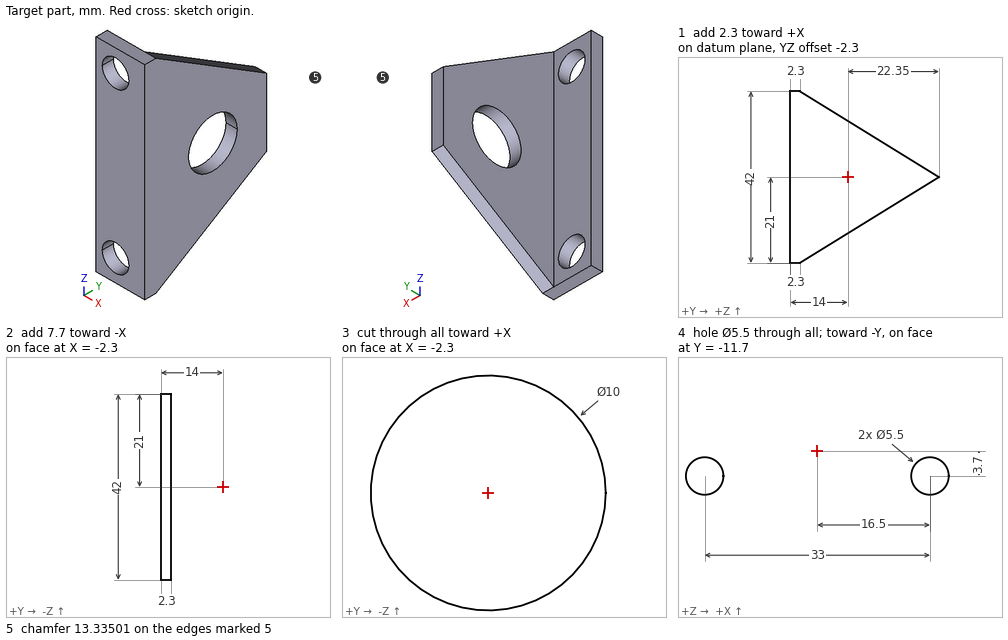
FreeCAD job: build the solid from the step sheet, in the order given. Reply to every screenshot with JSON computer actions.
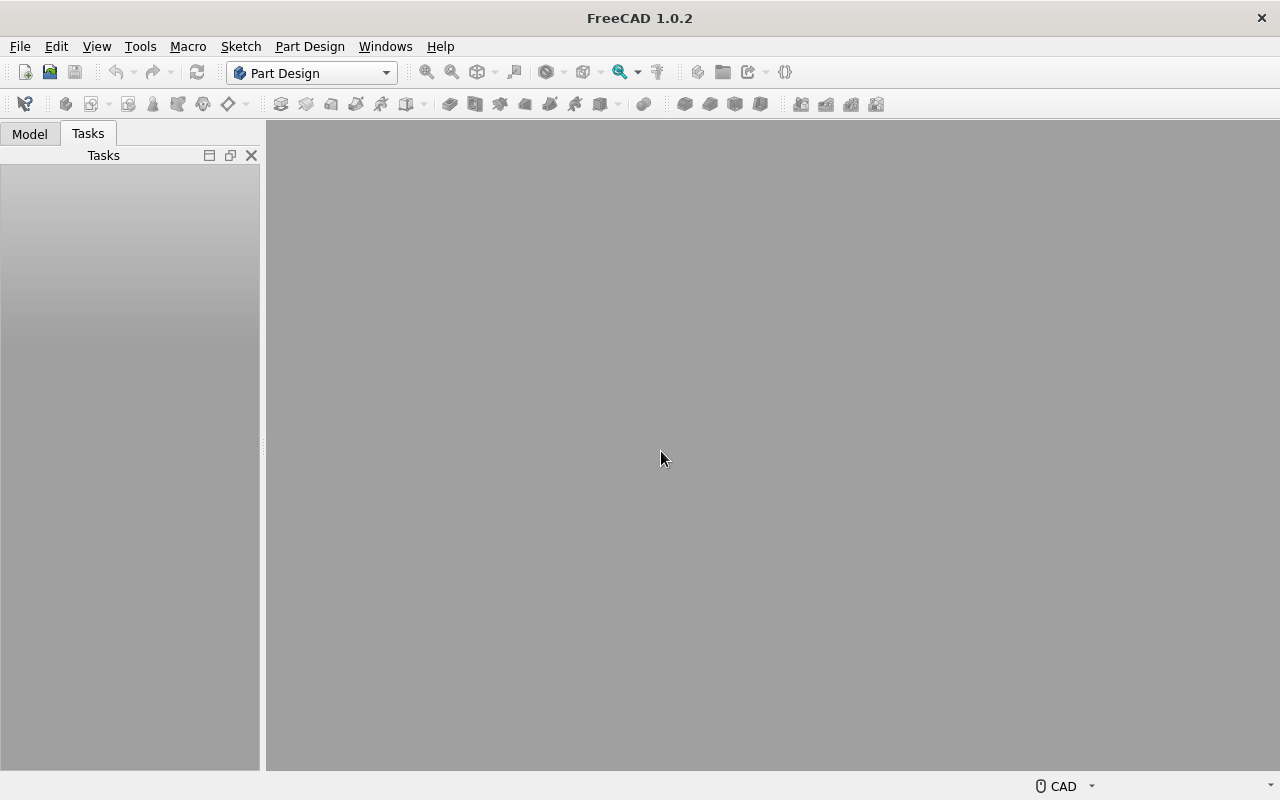
{"action": "key", "text": "ctrl+n"}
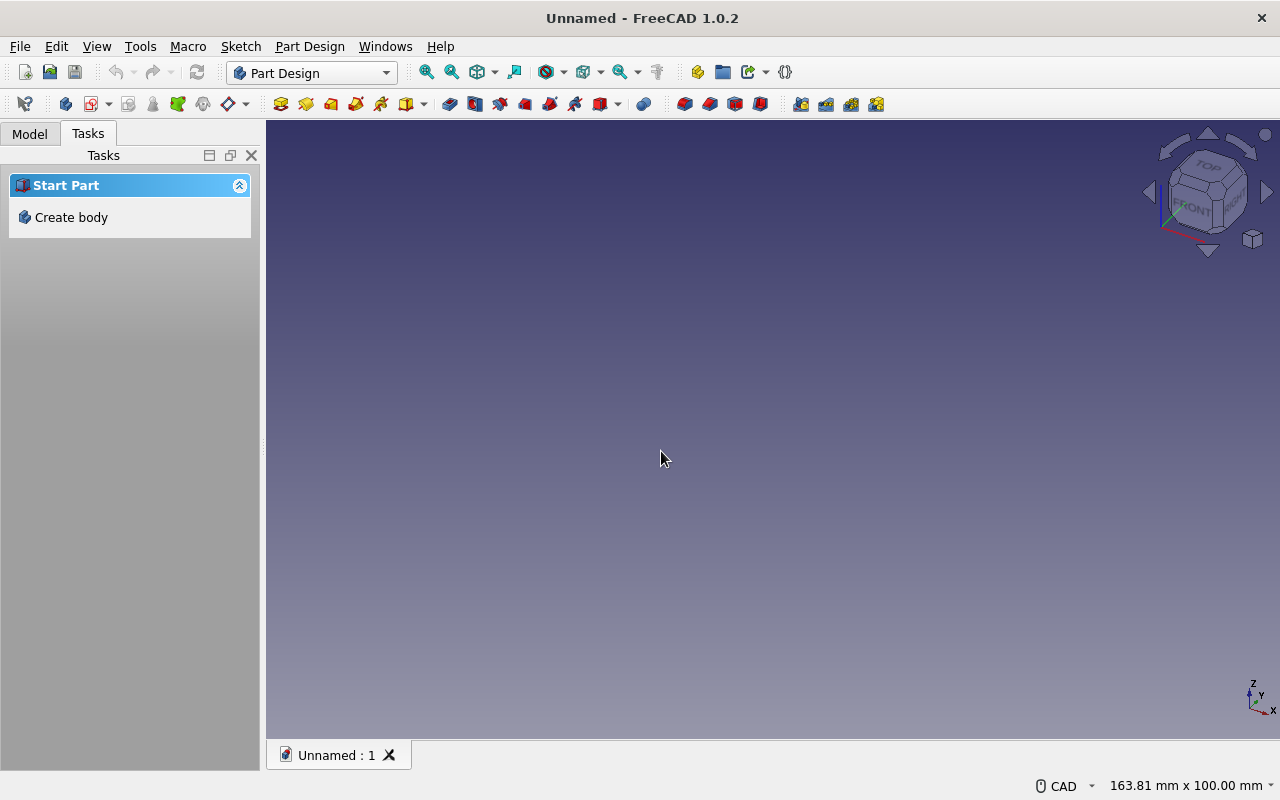
{"action": "left_click", "coordinate": [66, 104]}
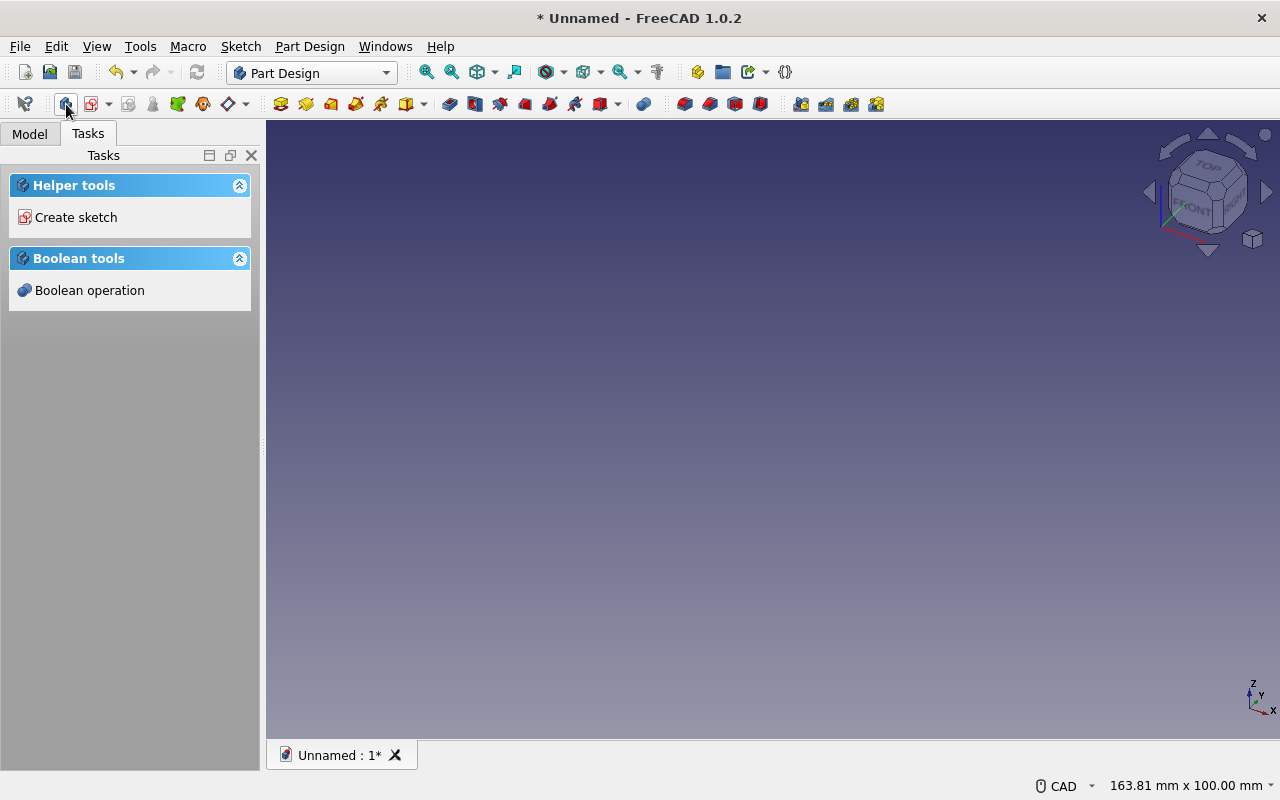
{"action": "left_click", "coordinate": [30, 134]}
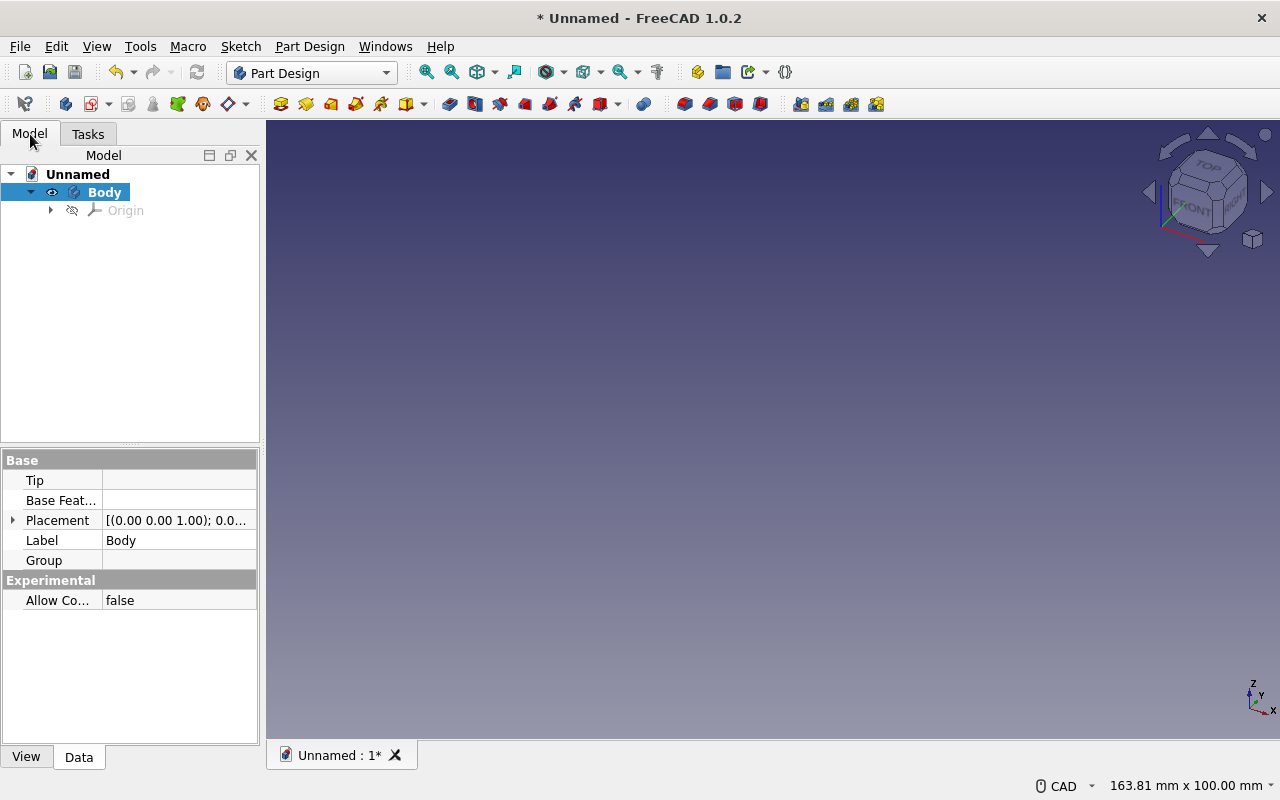
{"action": "left_click", "coordinate": [51, 210]}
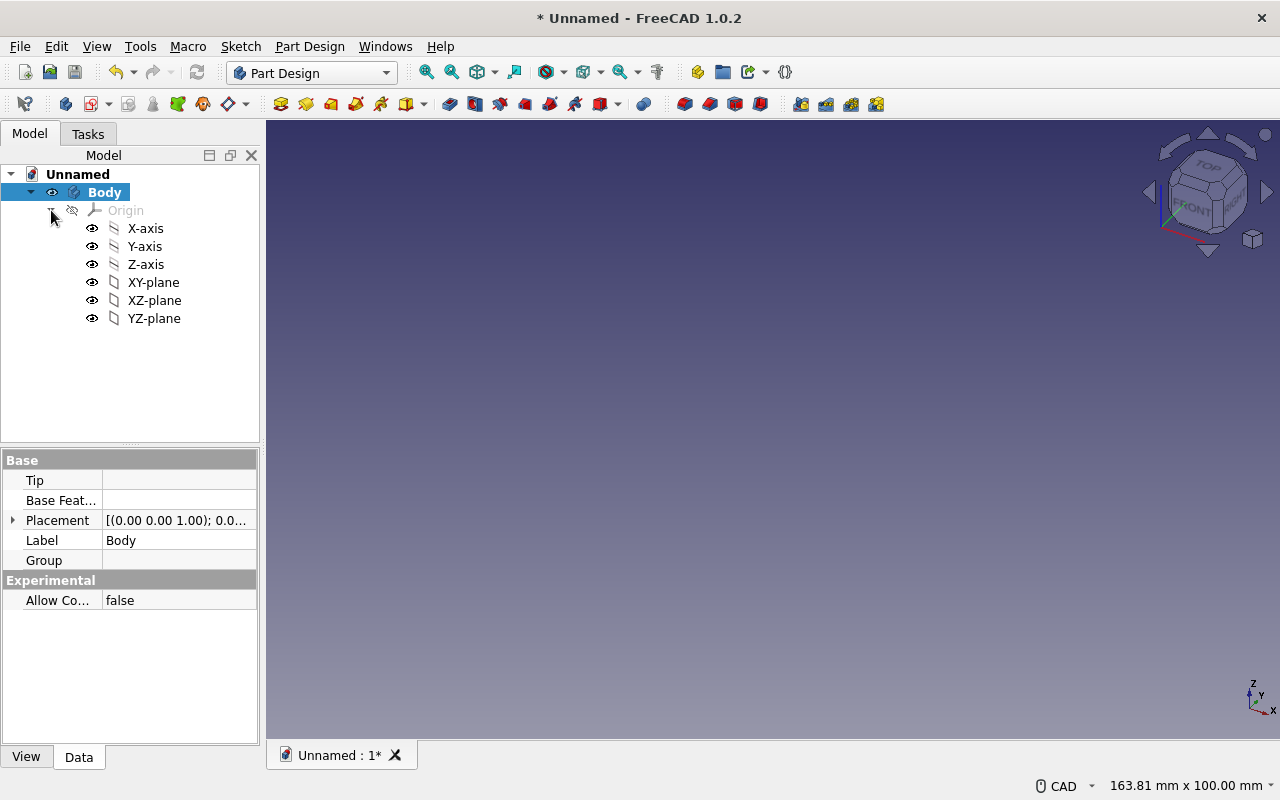
{"action": "left_click", "coordinate": [137, 318]}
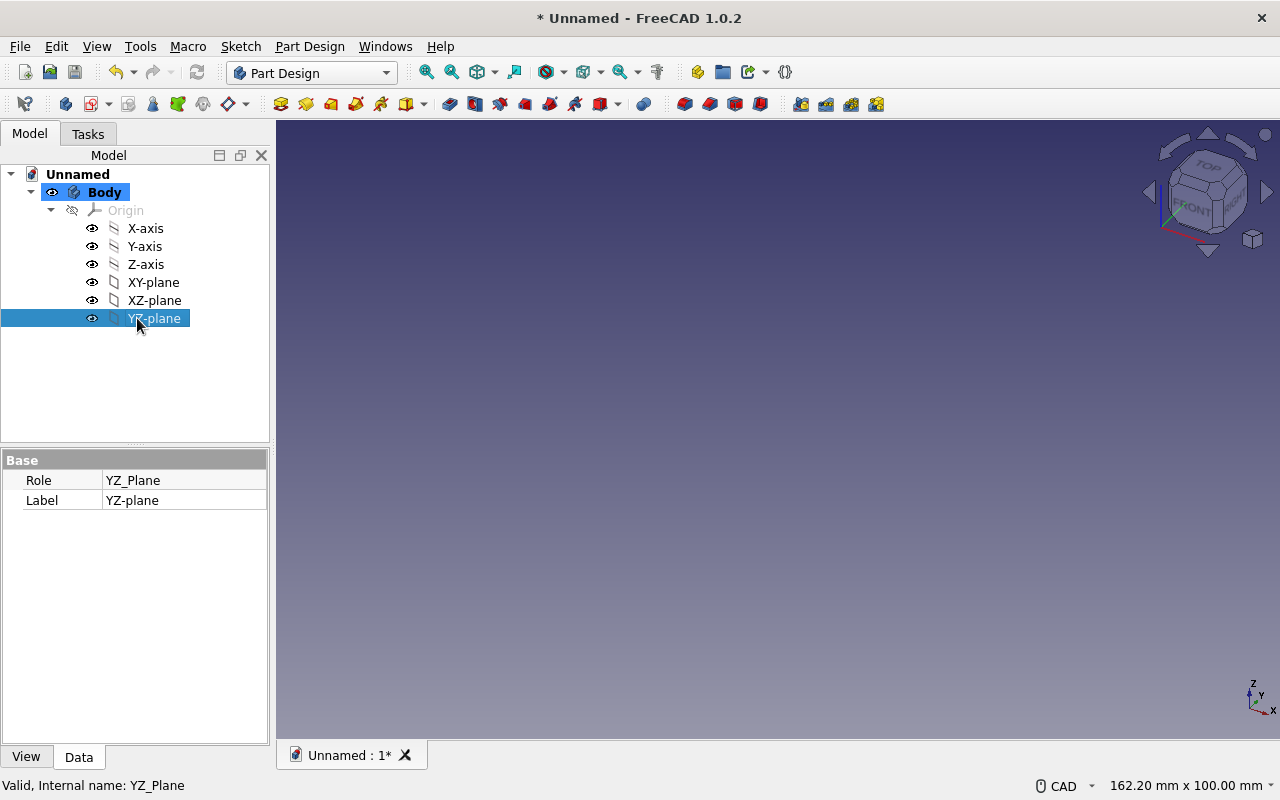
{"action": "left_click", "coordinate": [228, 104]}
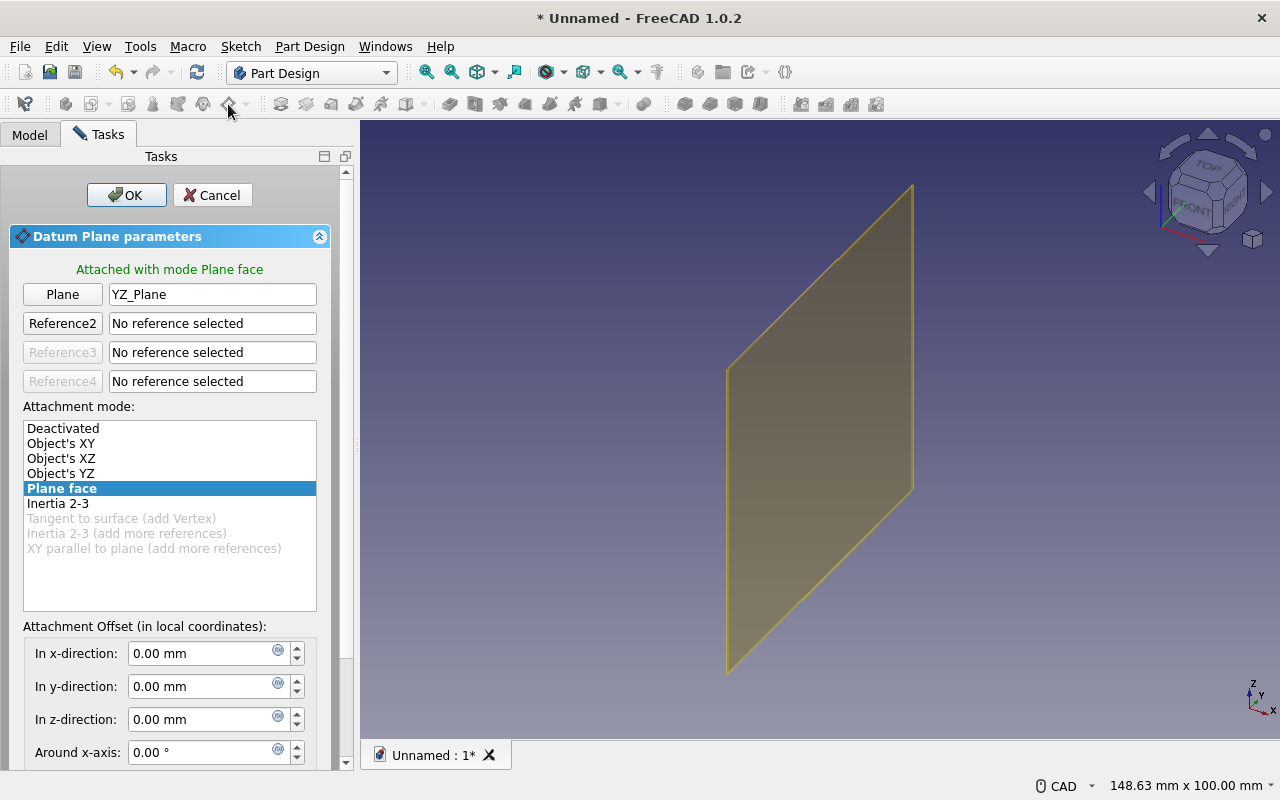
{"action": "triple_click", "coordinate": [210, 720]}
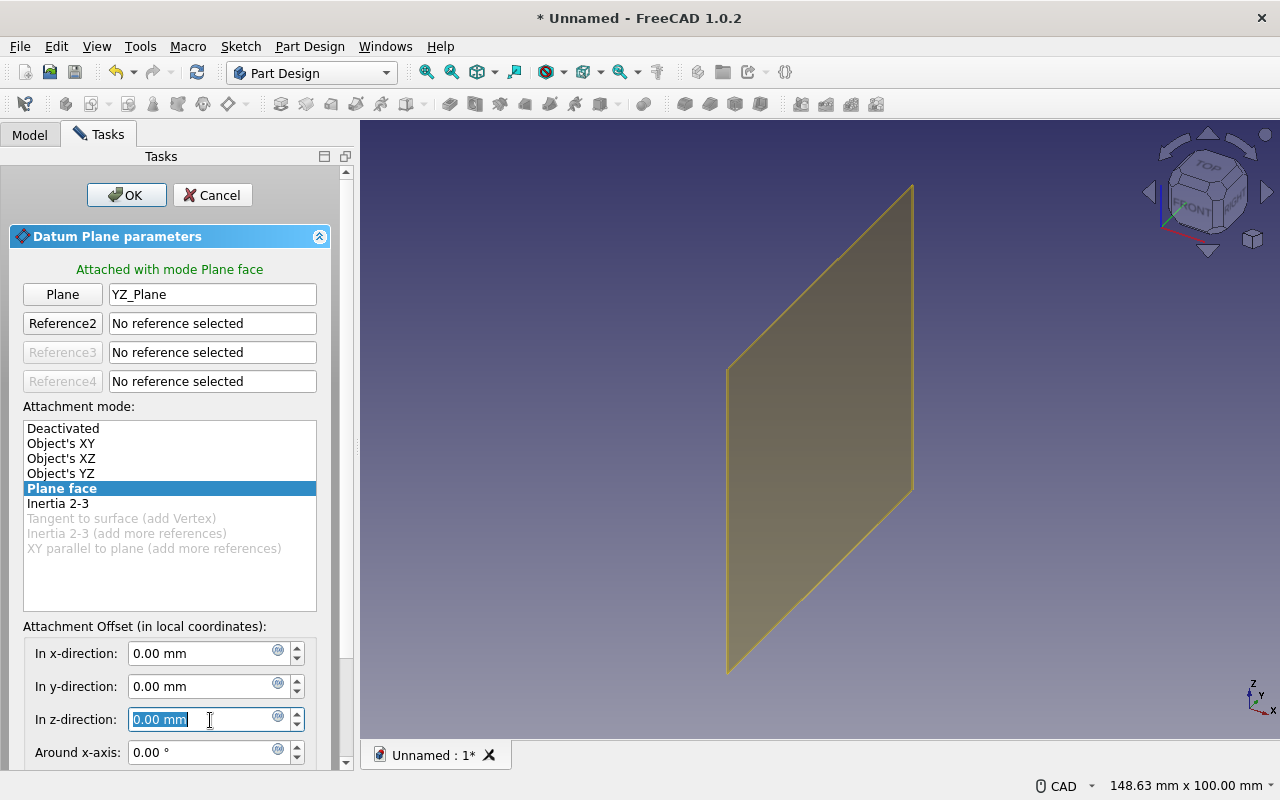
{"action": "type", "text": "-2.3"}
{"action": "key", "text": "Tab"}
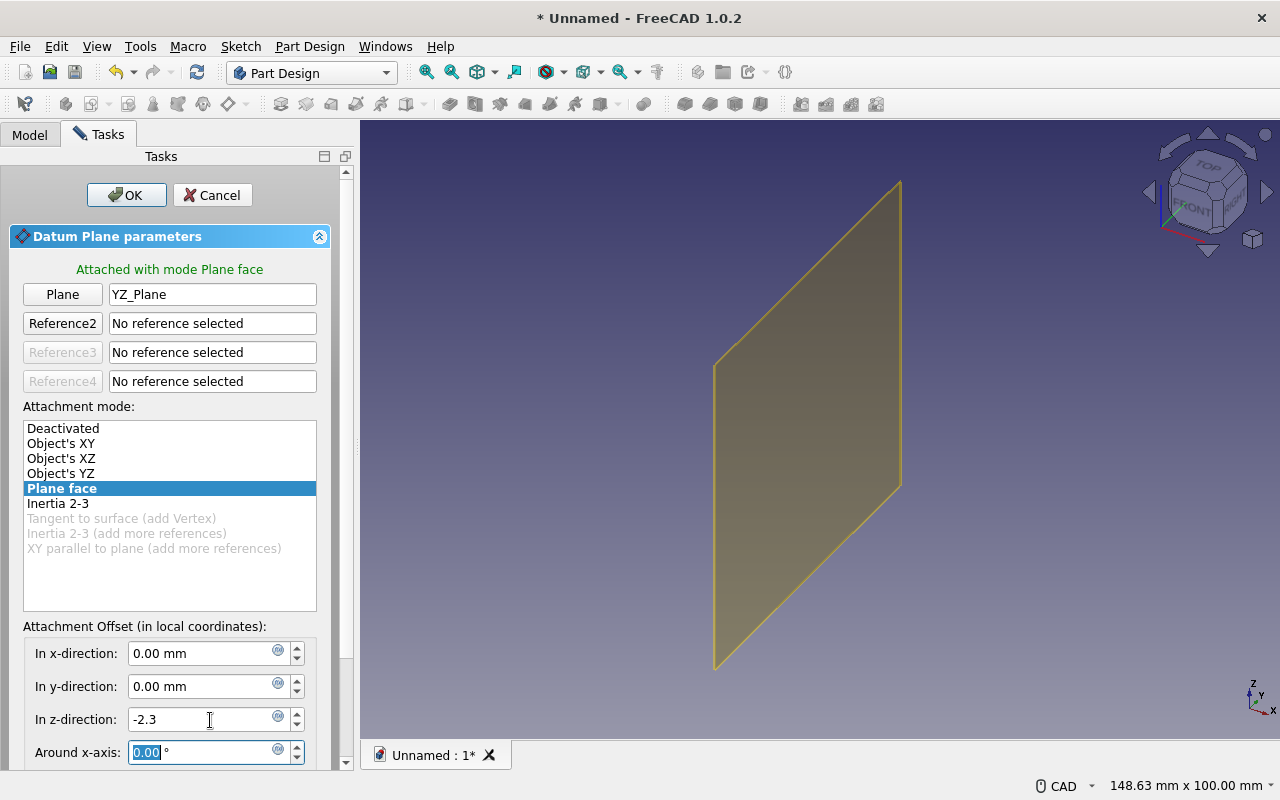
{"action": "left_click", "coordinate": [127, 195]}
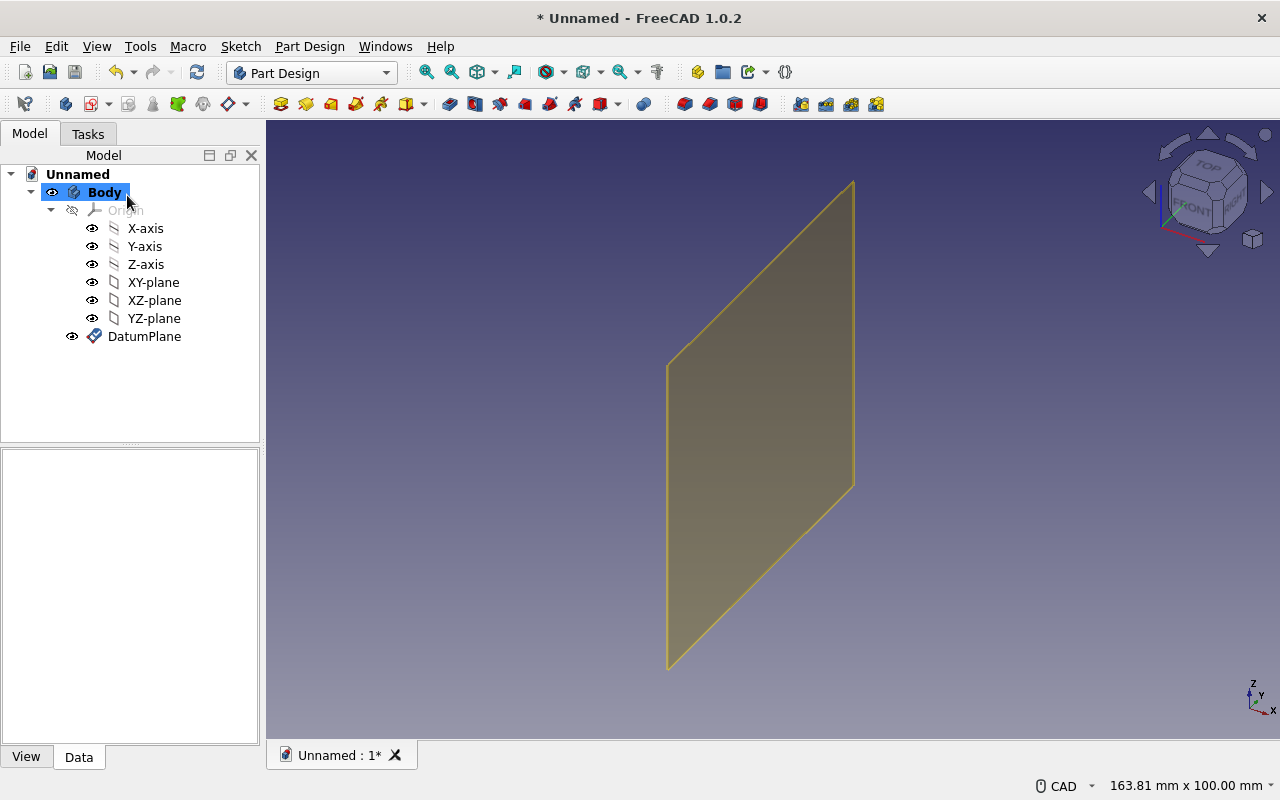
{"action": "left_click", "coordinate": [117, 336]}